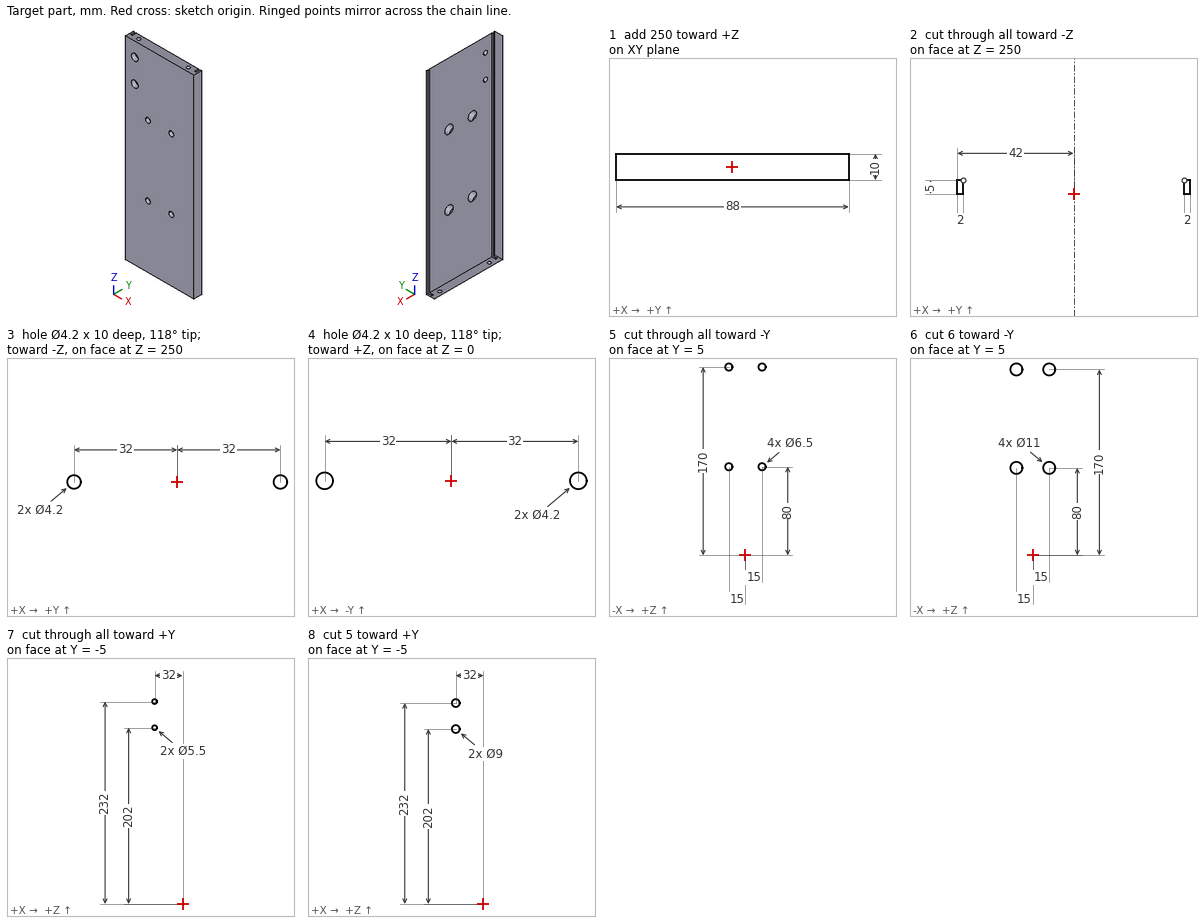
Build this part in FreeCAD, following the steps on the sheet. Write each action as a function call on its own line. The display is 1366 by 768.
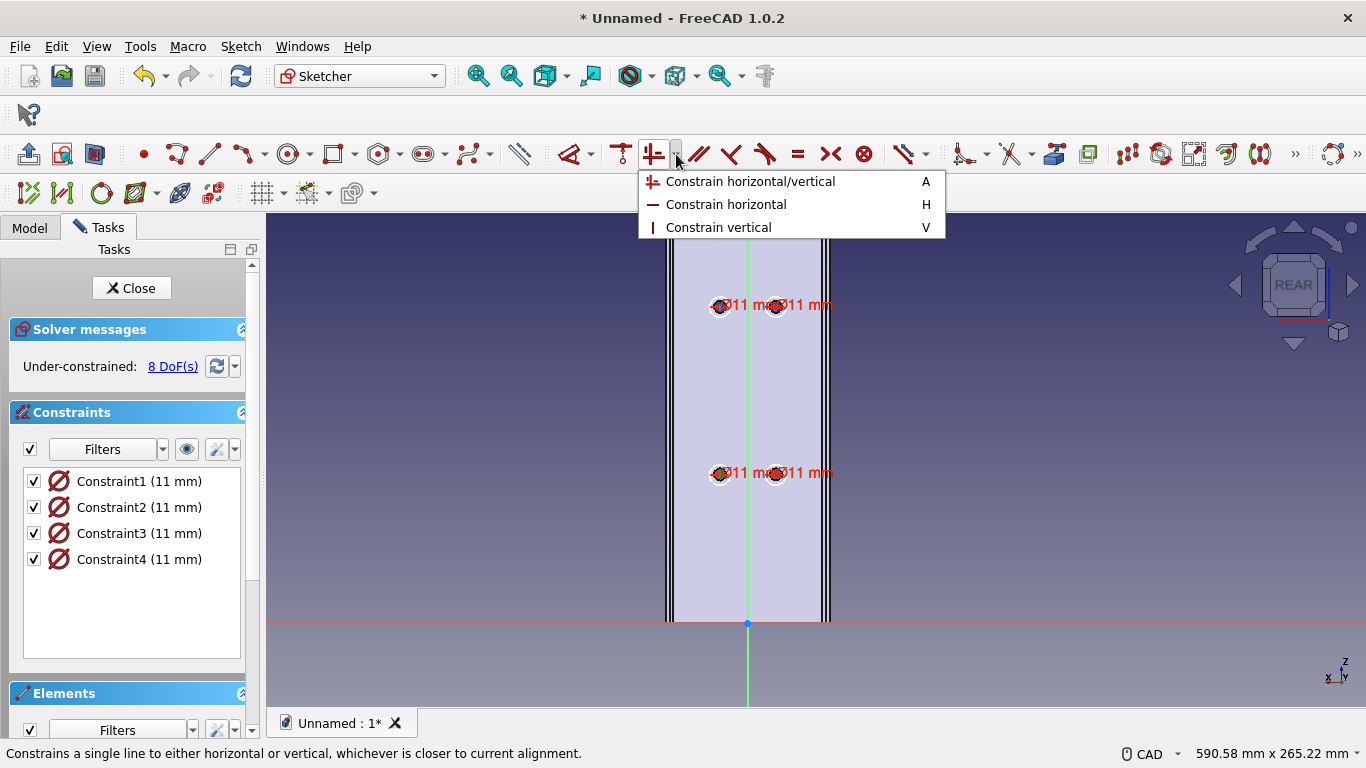
click(792, 204)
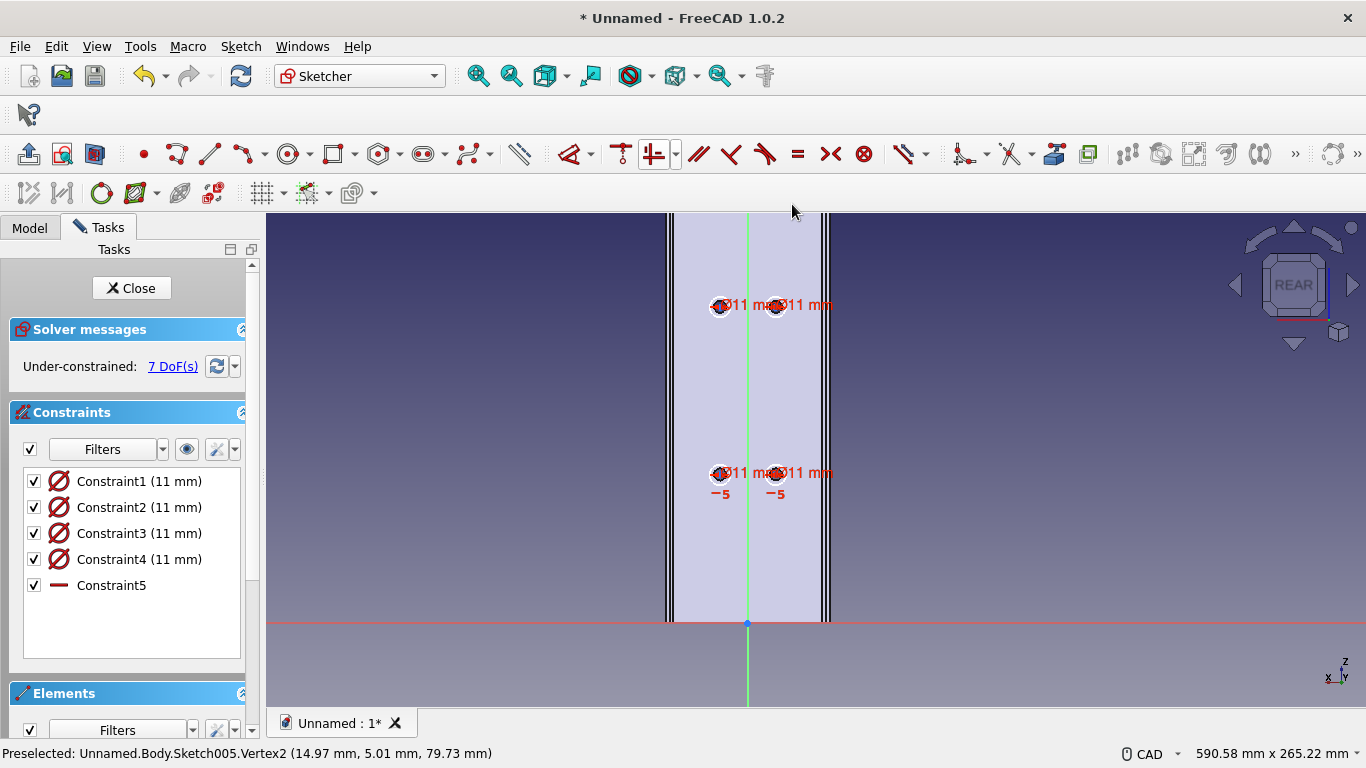
click(776, 475)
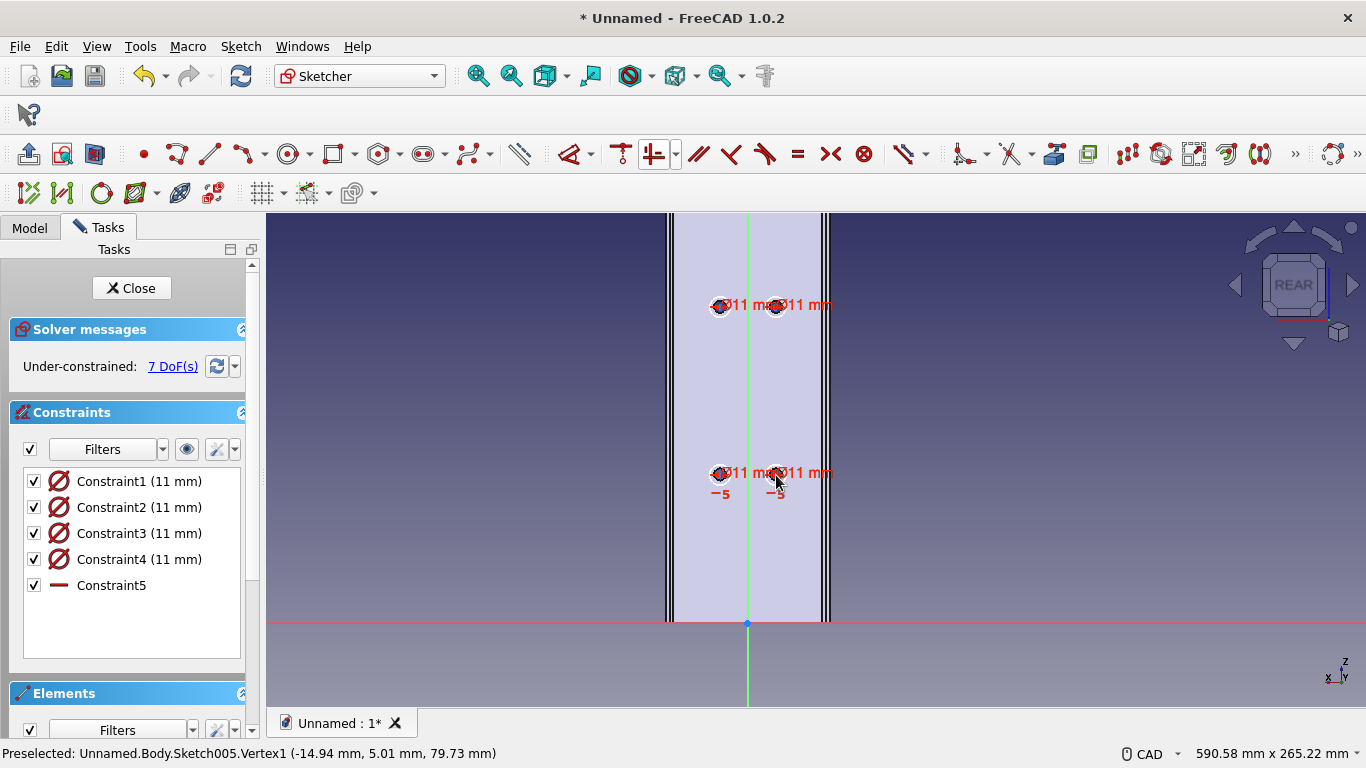
click(776, 307)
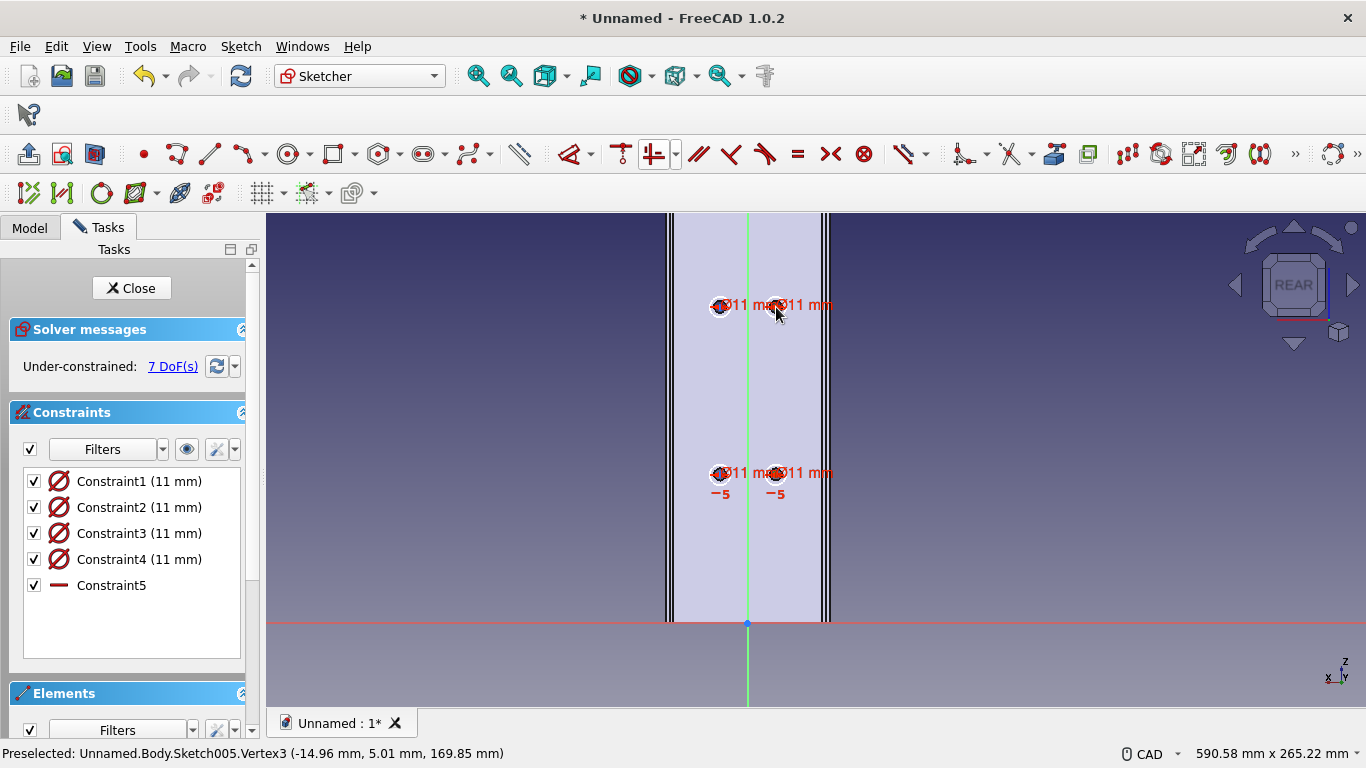
click(676, 154)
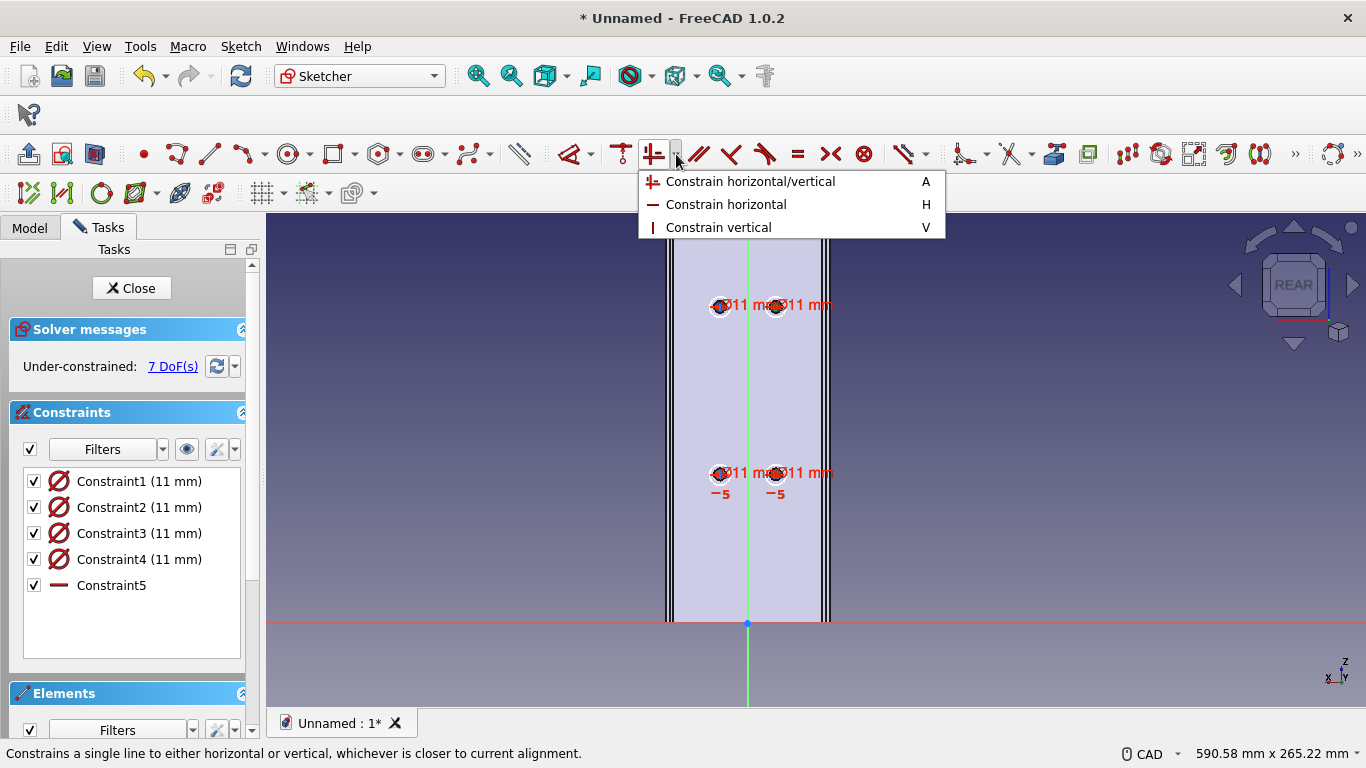
click(792, 228)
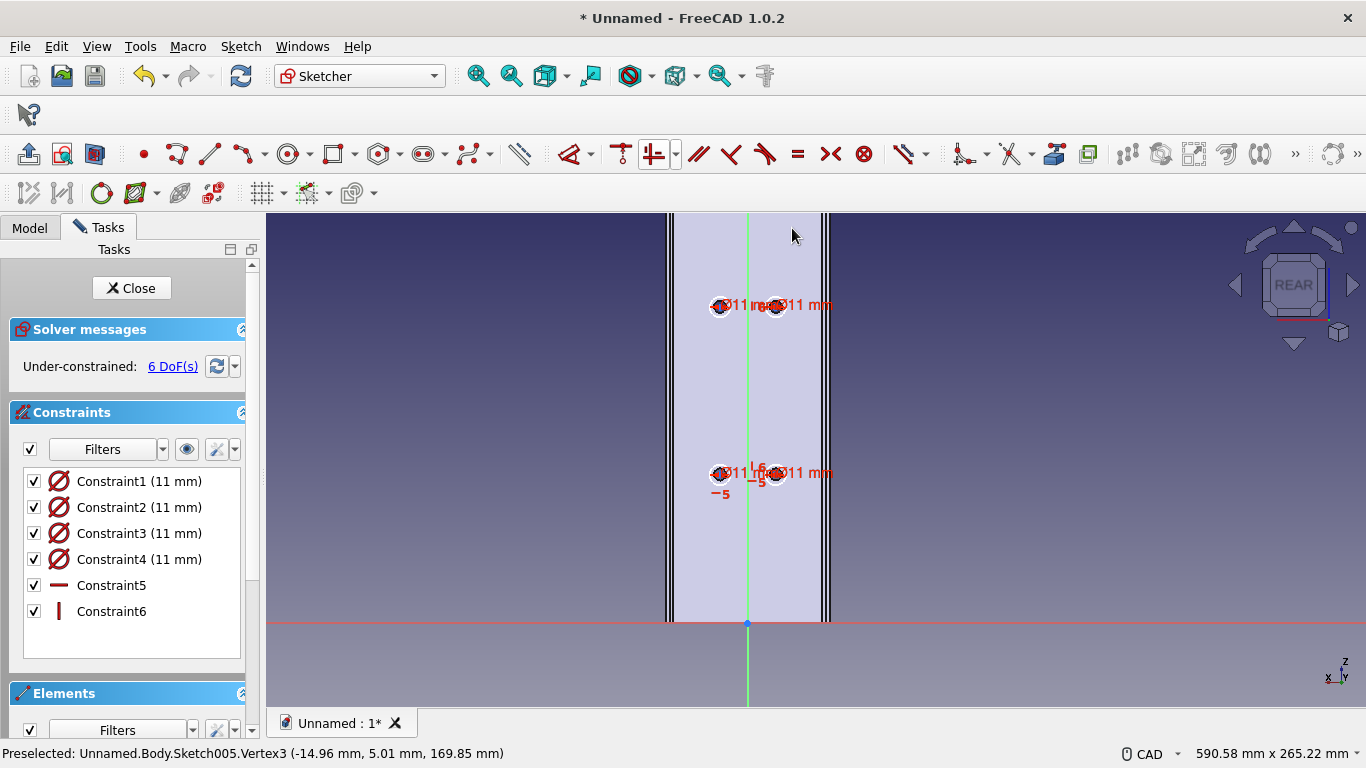
click(720, 475)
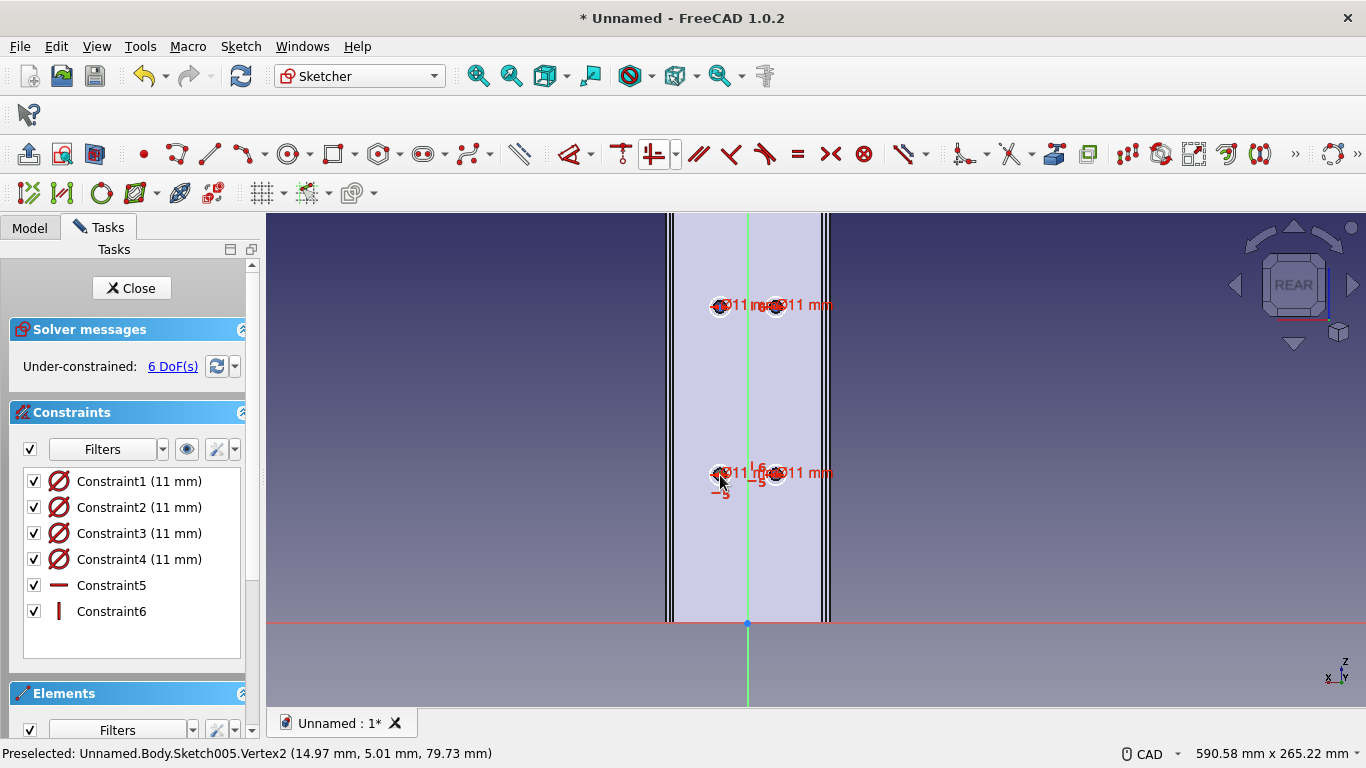
click(720, 307)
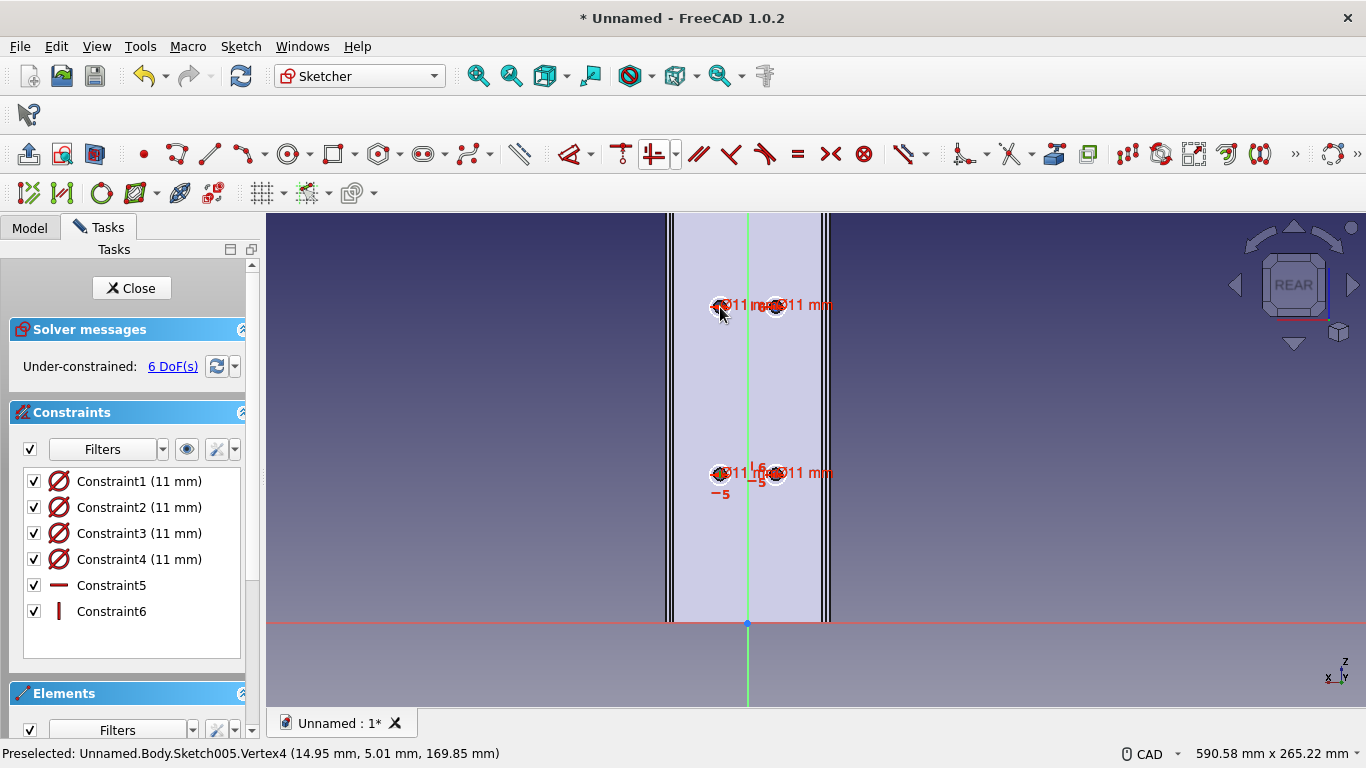
key(v)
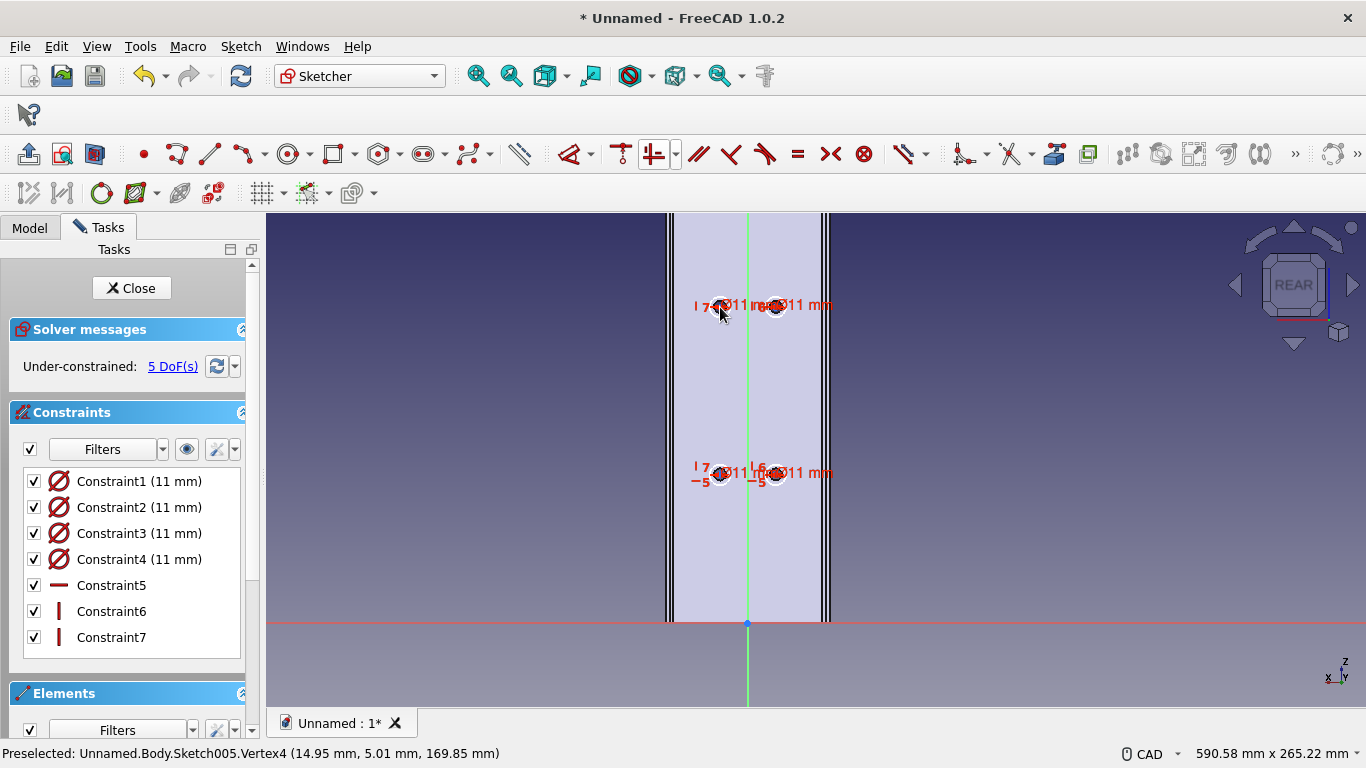
click(776, 307)